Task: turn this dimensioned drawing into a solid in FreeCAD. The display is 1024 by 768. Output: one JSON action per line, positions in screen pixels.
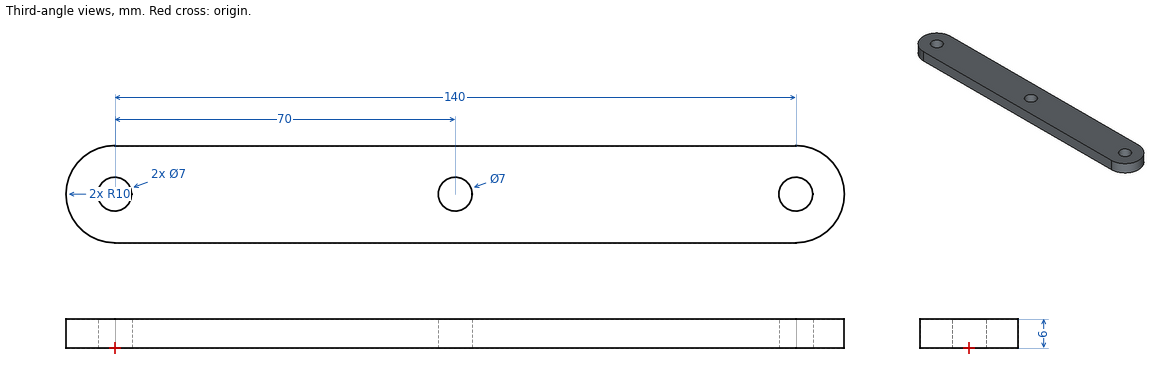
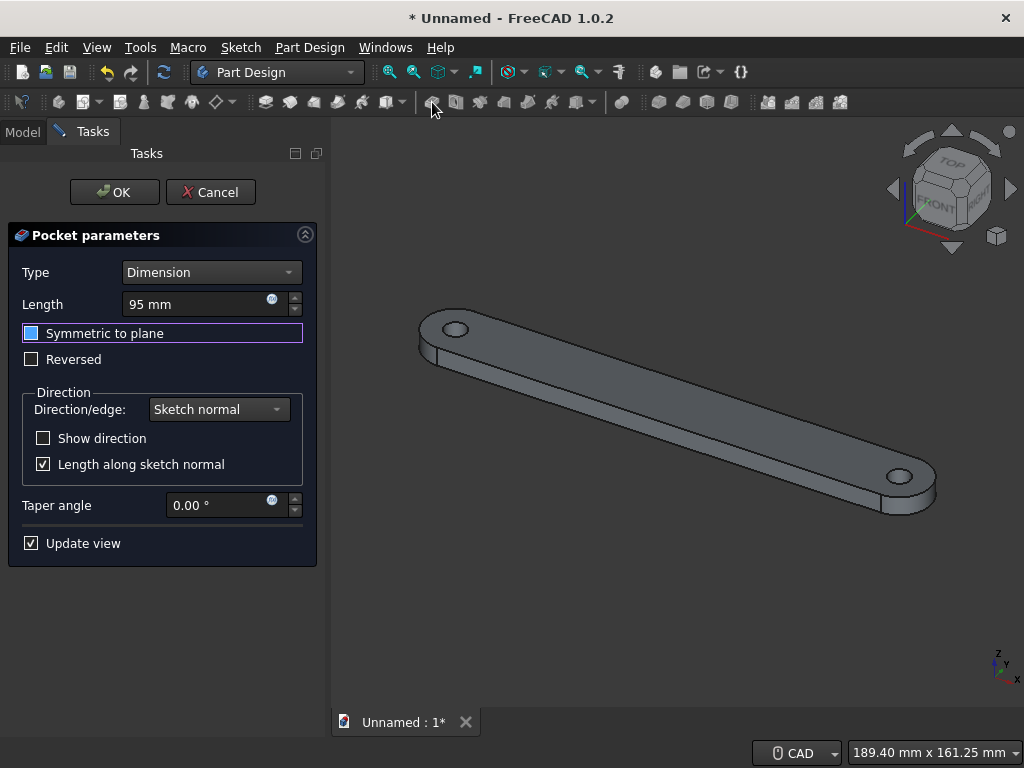
{"action": "left_click", "coordinate": [115, 192]}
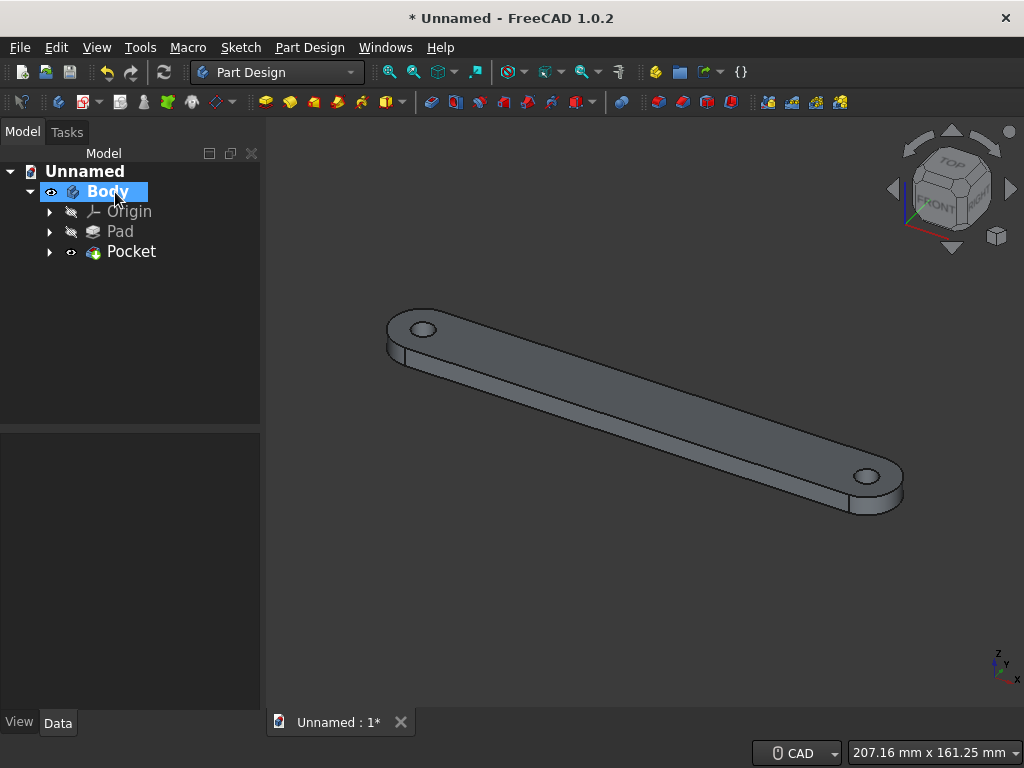
{"action": "left_click", "coordinate": [790, 450]}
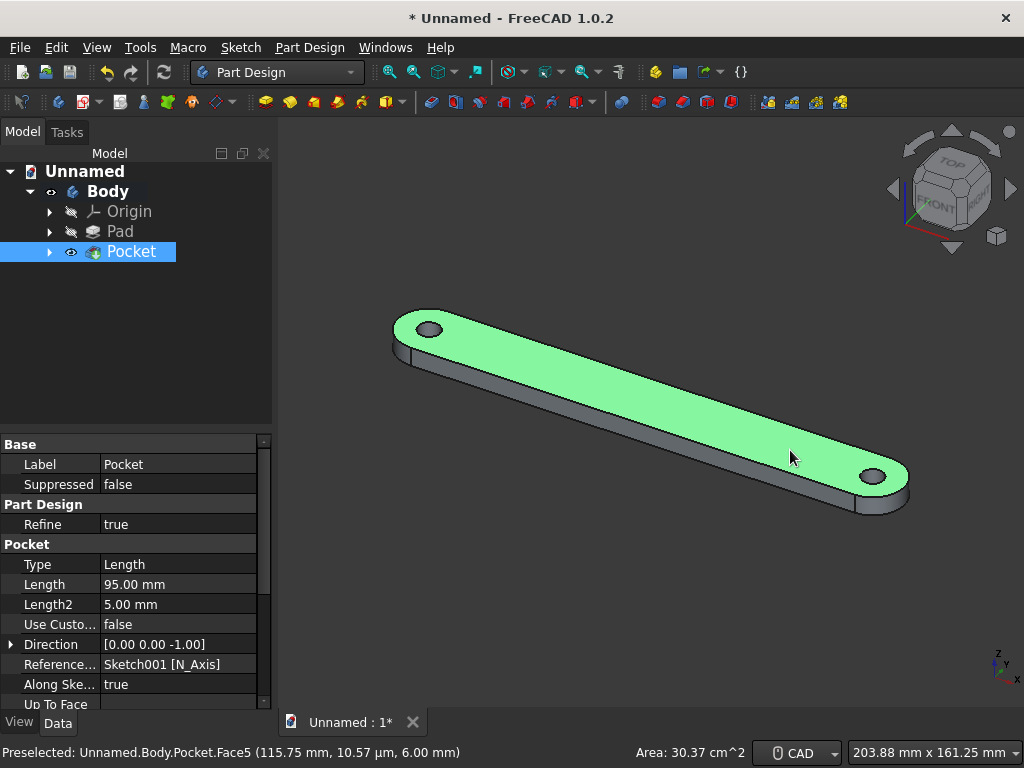
{"action": "left_click", "coordinate": [84, 102]}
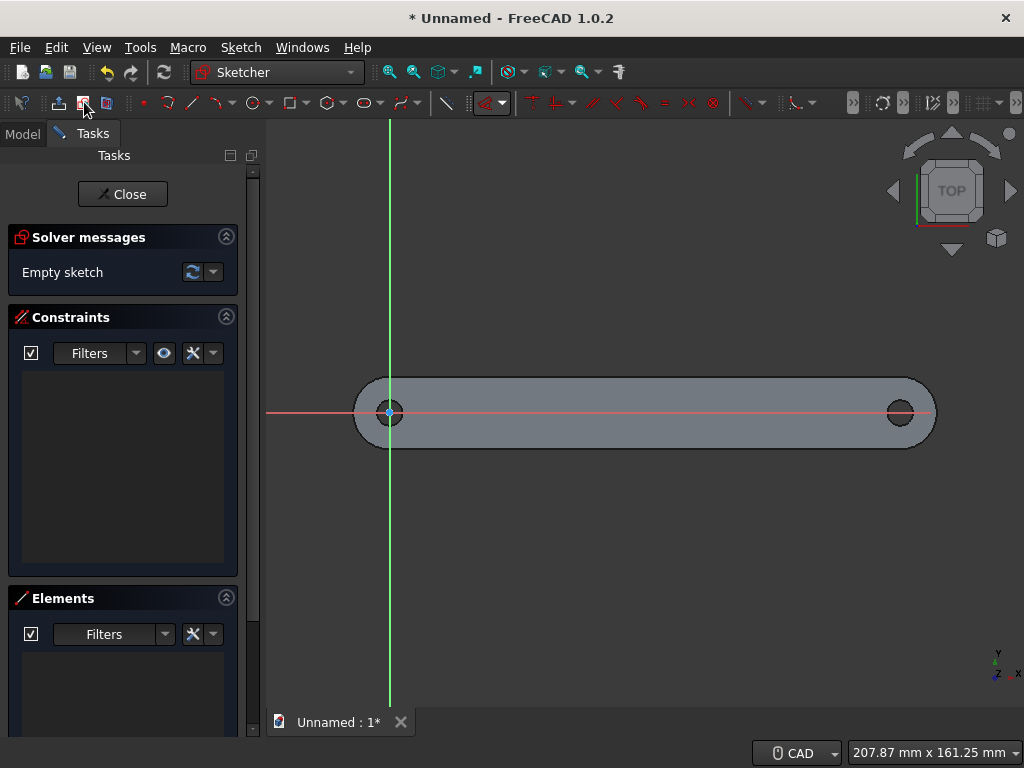
{"action": "scroll", "coordinate": [650, 413], "scroll_direction": "up", "scroll_amount": 13}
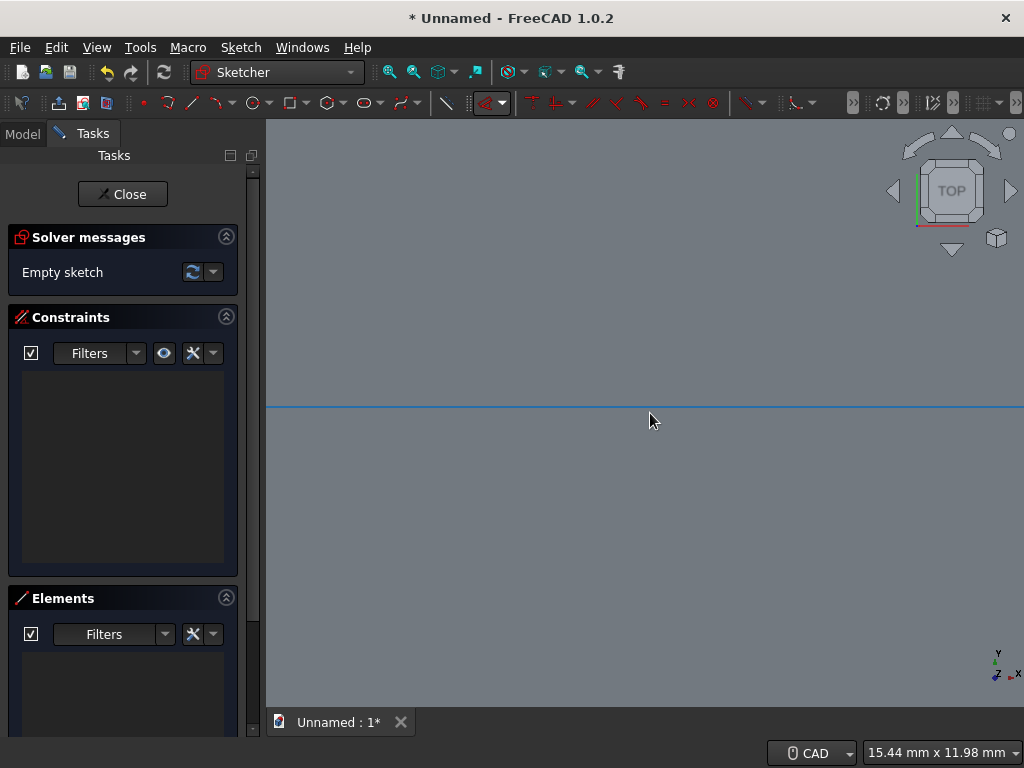
{"action": "left_click", "coordinate": [254, 104]}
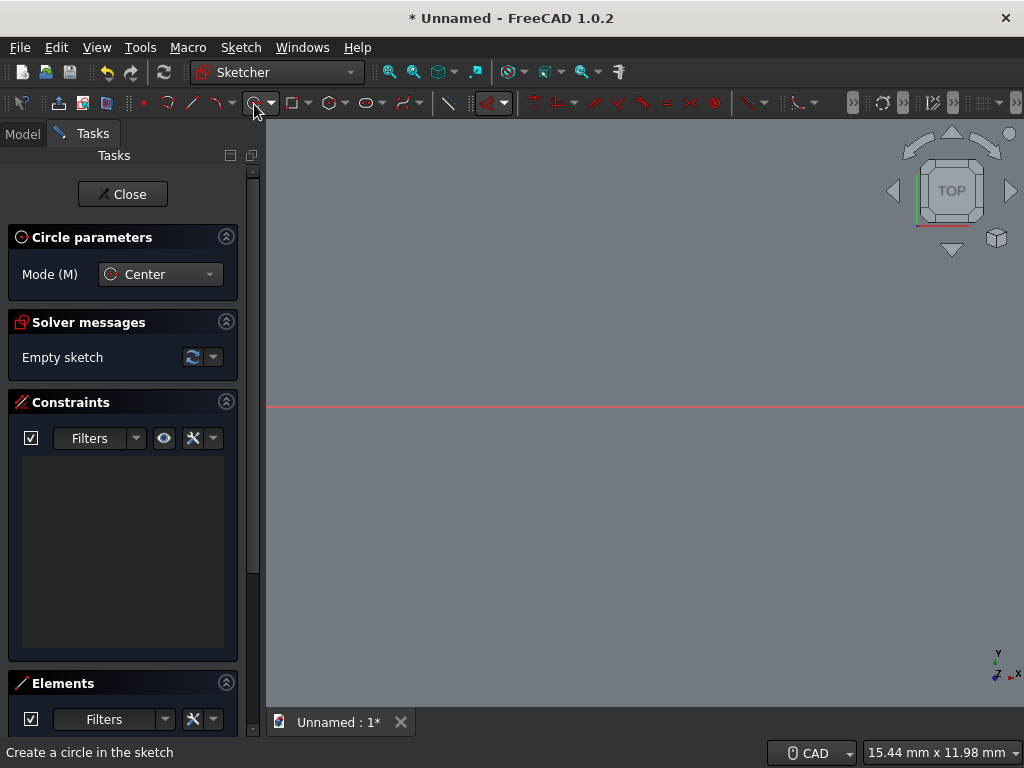
{"action": "left_click", "coordinate": [576, 407]}
{"action": "mouse_move", "coordinate": [698, 285]}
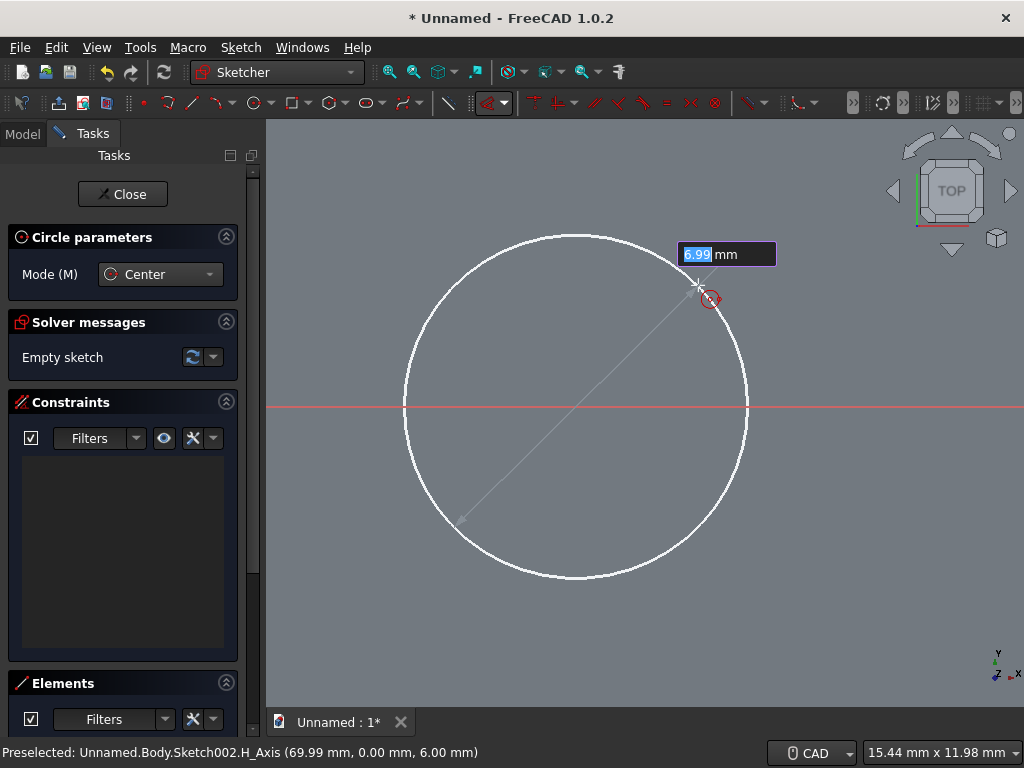
{"action": "type", "text": "7"}
{"action": "key", "text": "Return"}
{"action": "key", "text": "Escape"}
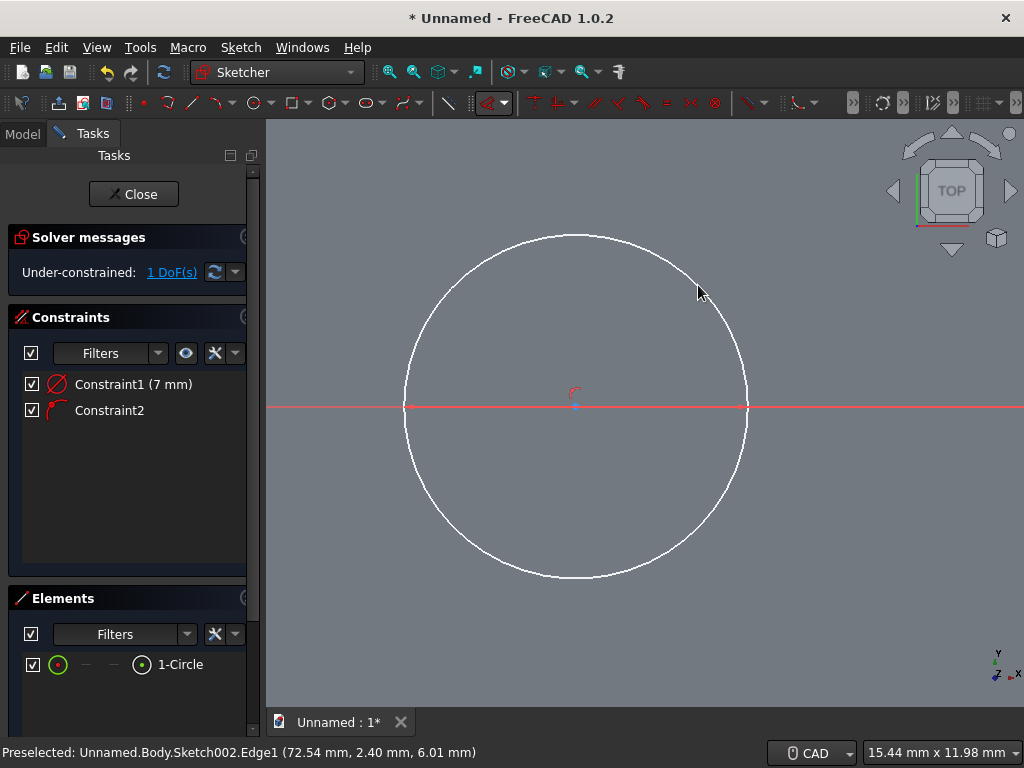
{"action": "left_click", "coordinate": [576, 407]}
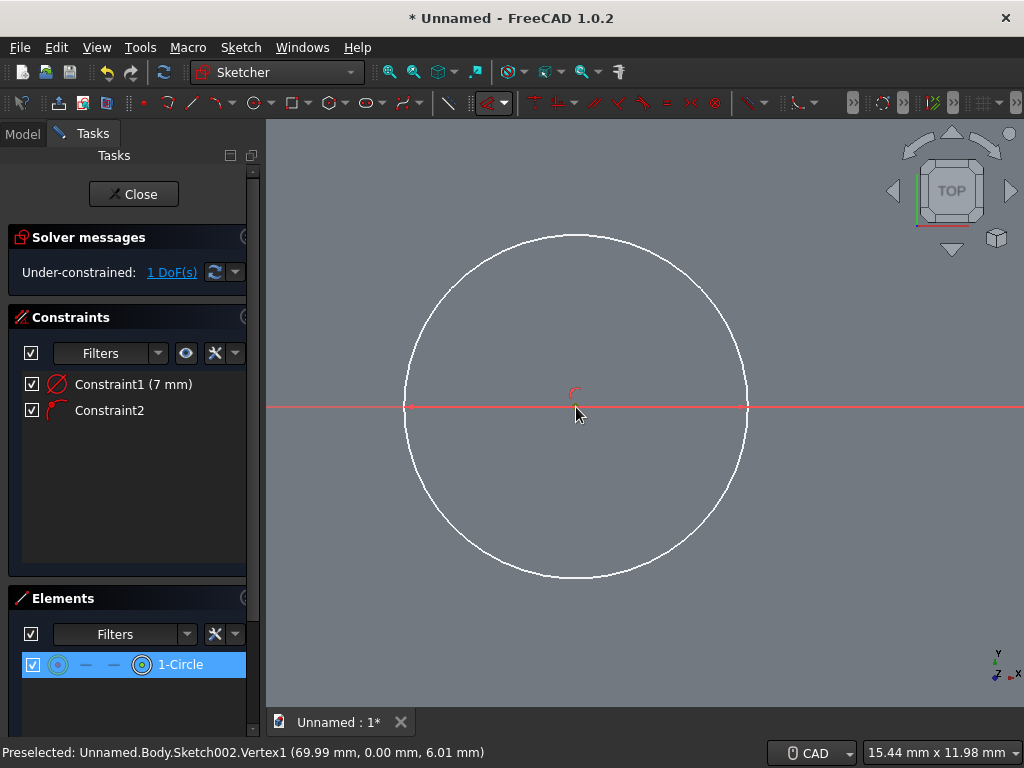
{"action": "left_click", "coordinate": [506, 104]}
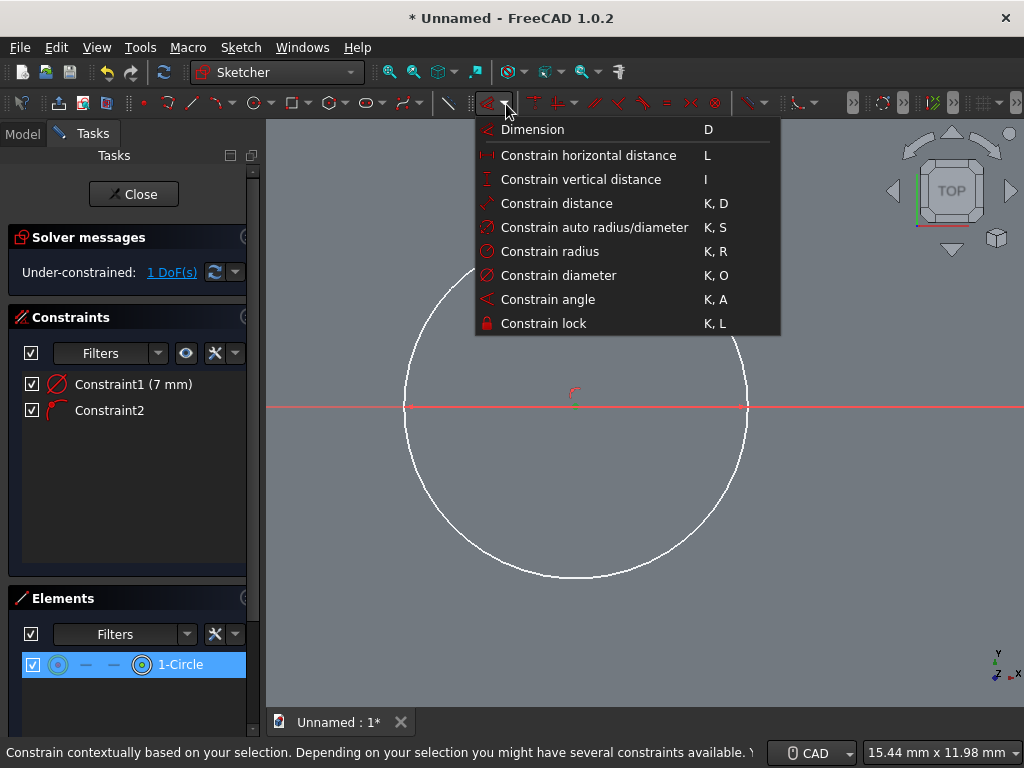
{"action": "left_click", "coordinate": [628, 155]}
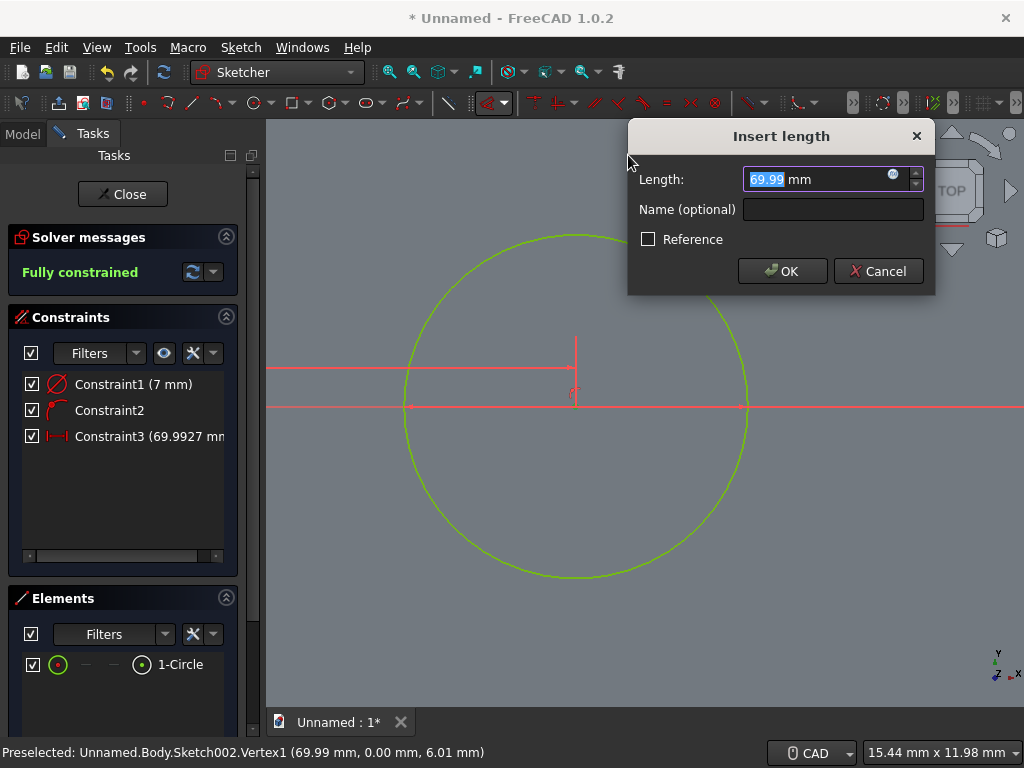
{"action": "type", "text": "70"}
{"action": "key", "text": "Return"}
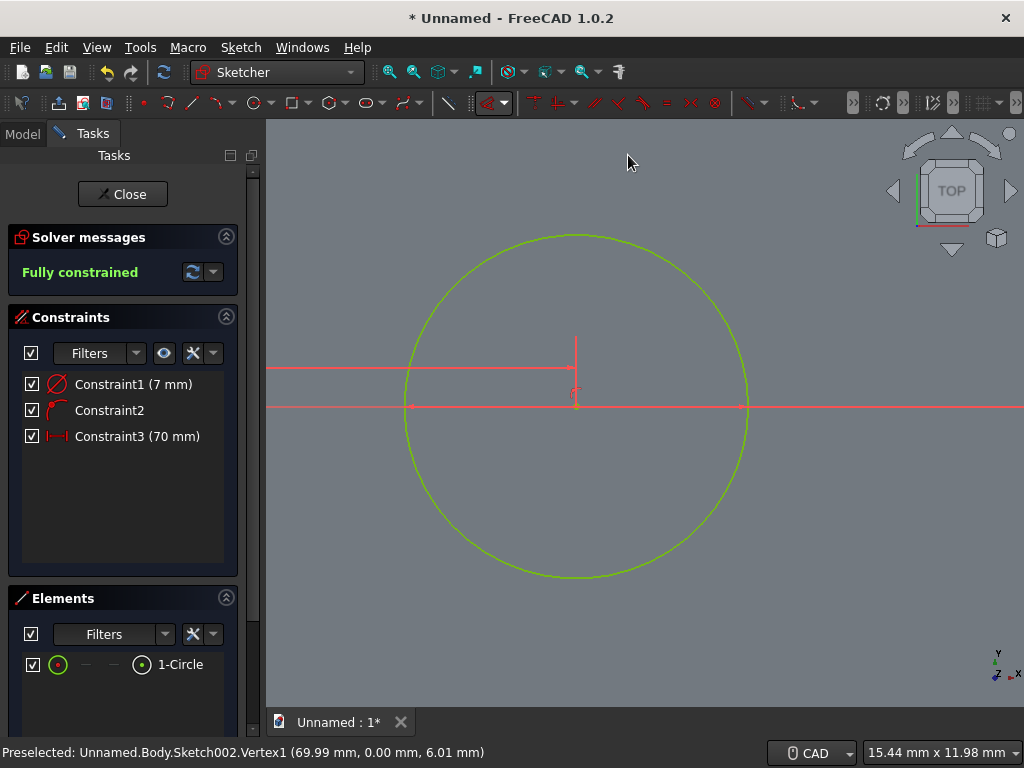
{"action": "left_click", "coordinate": [123, 194]}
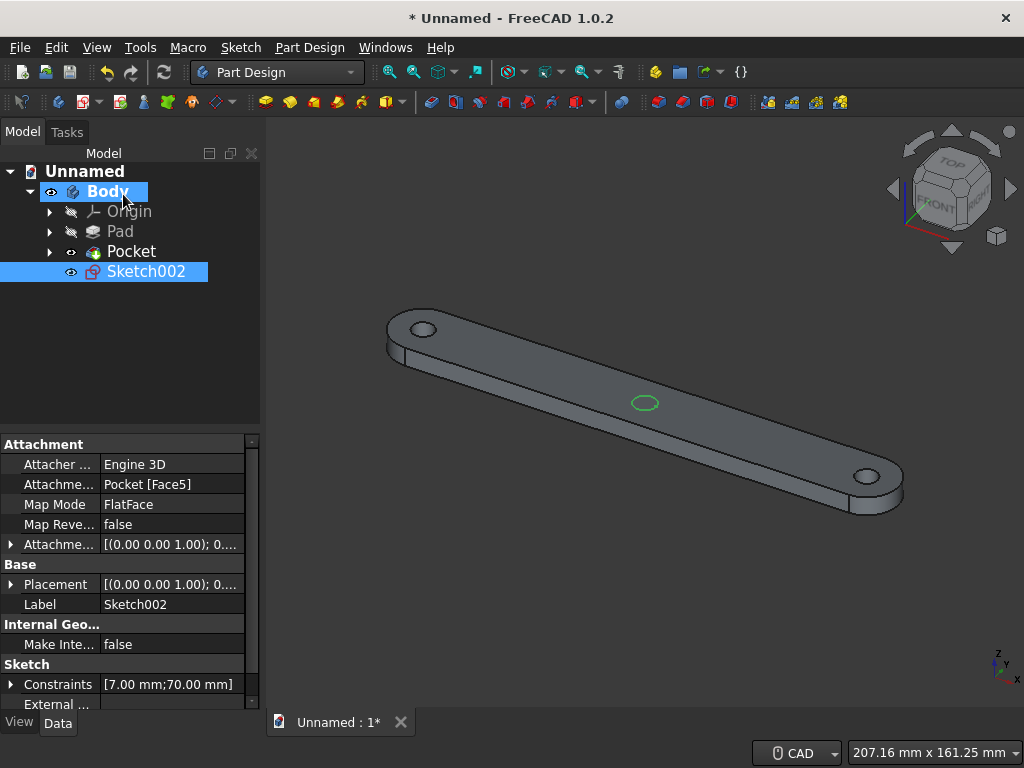
{"action": "left_click", "coordinate": [432, 102]}